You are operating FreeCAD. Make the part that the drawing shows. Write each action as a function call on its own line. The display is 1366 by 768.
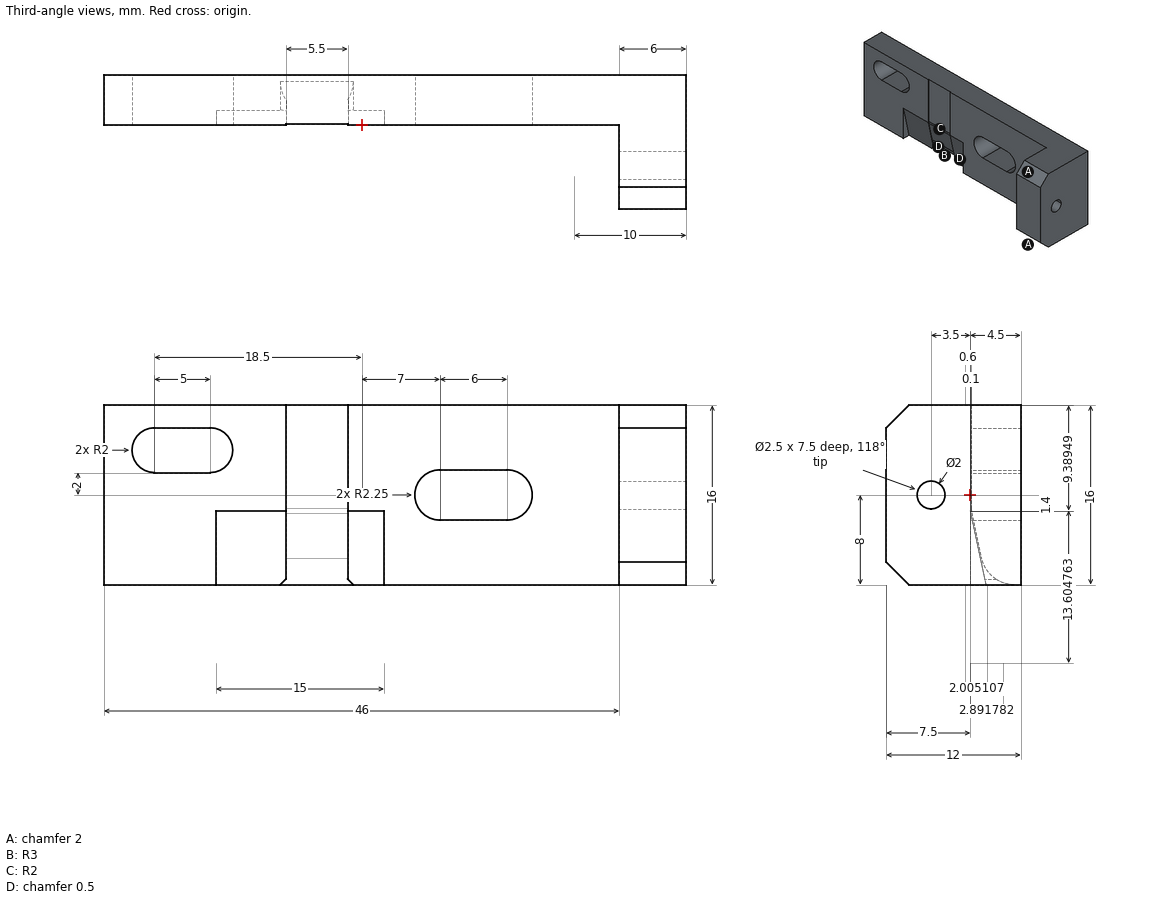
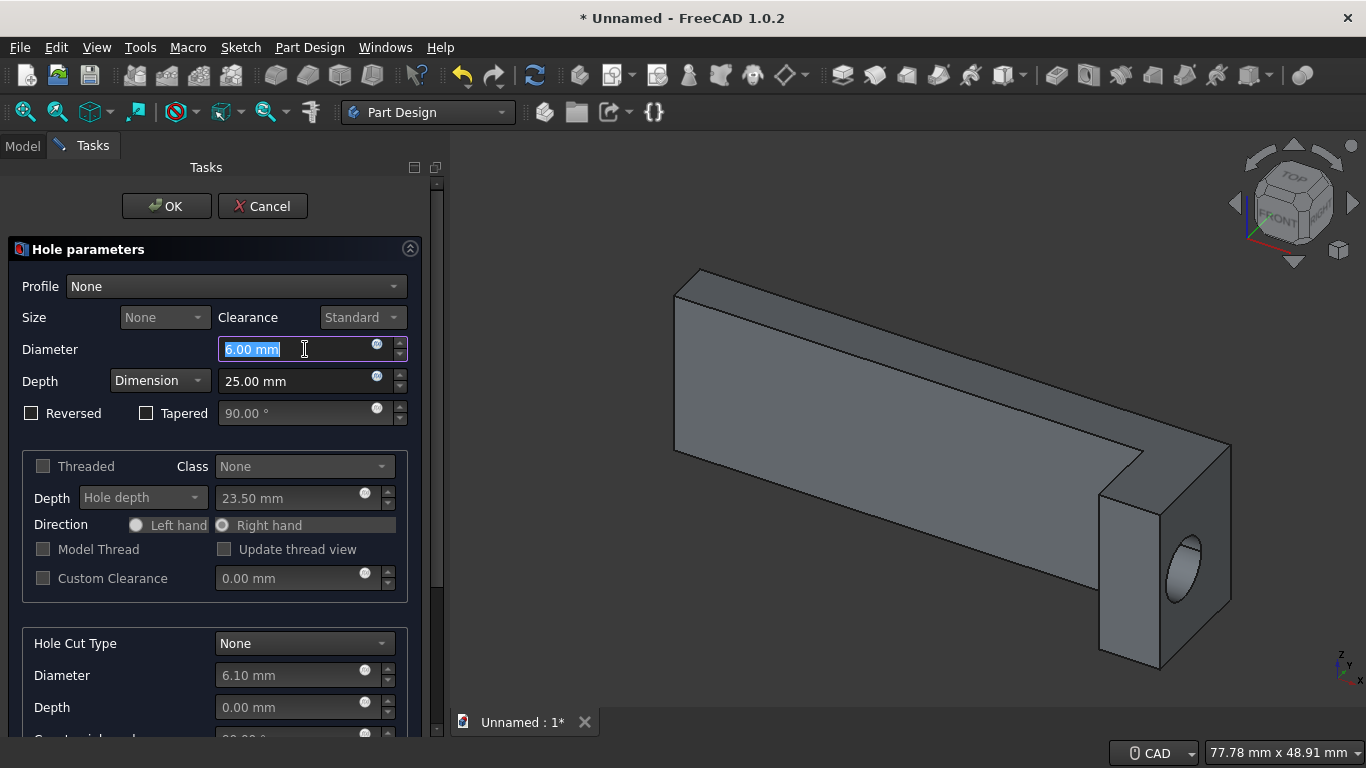
text(2.5)
key(Tab)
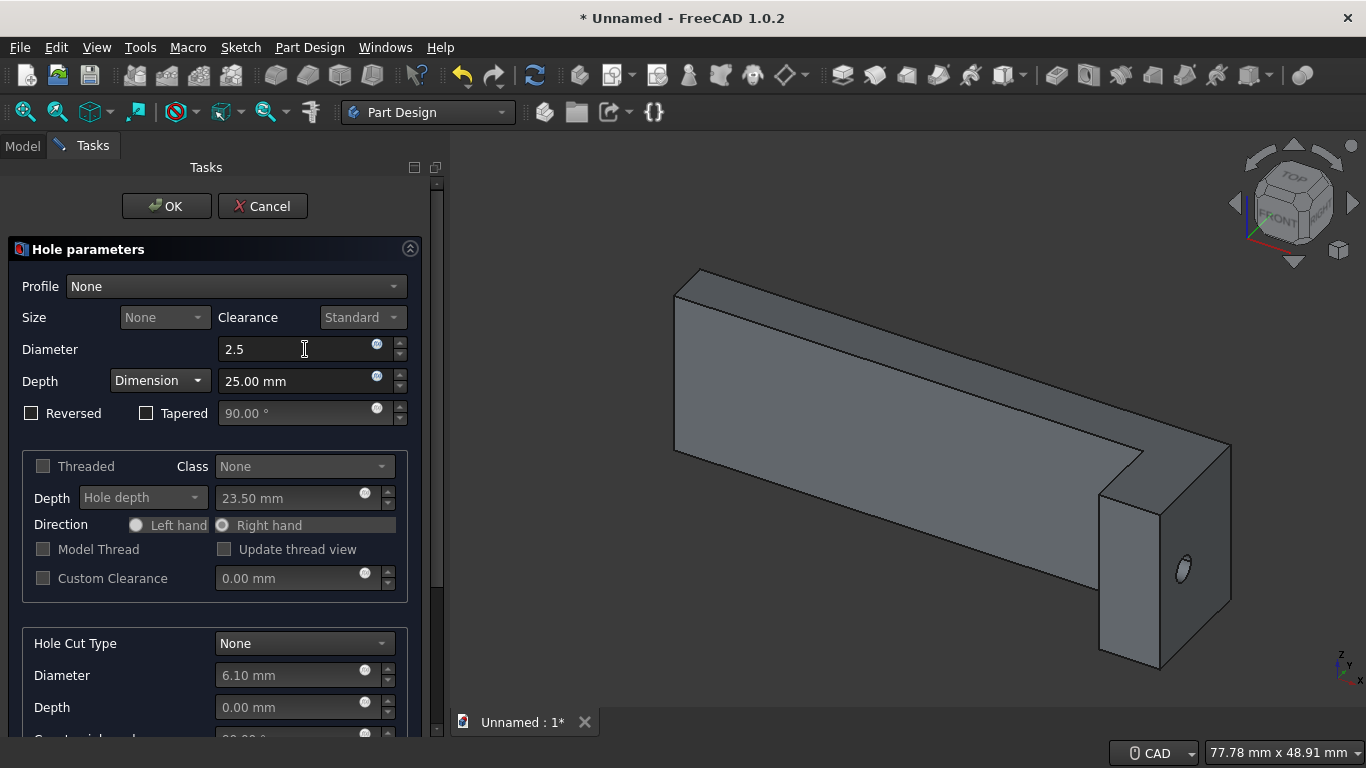
triple_click(305, 381)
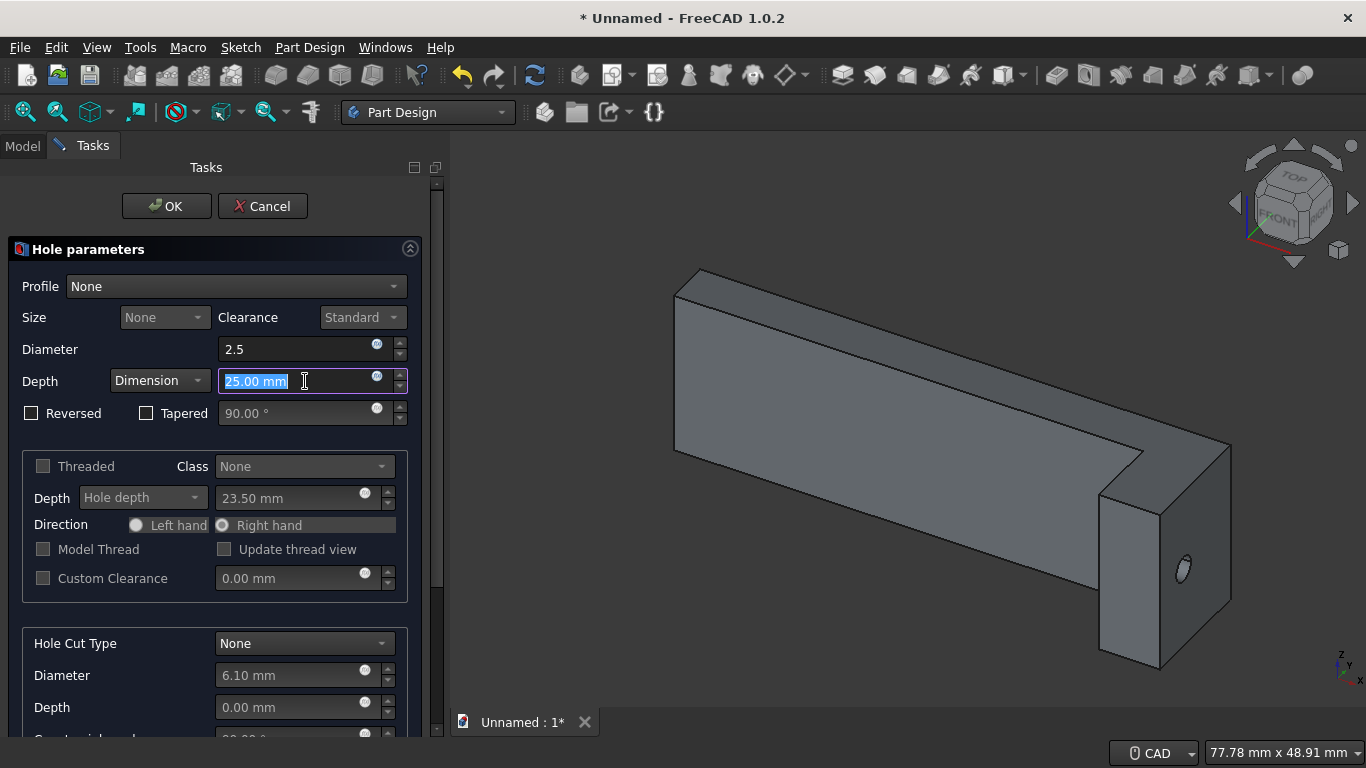
text(7.5)
key(Tab)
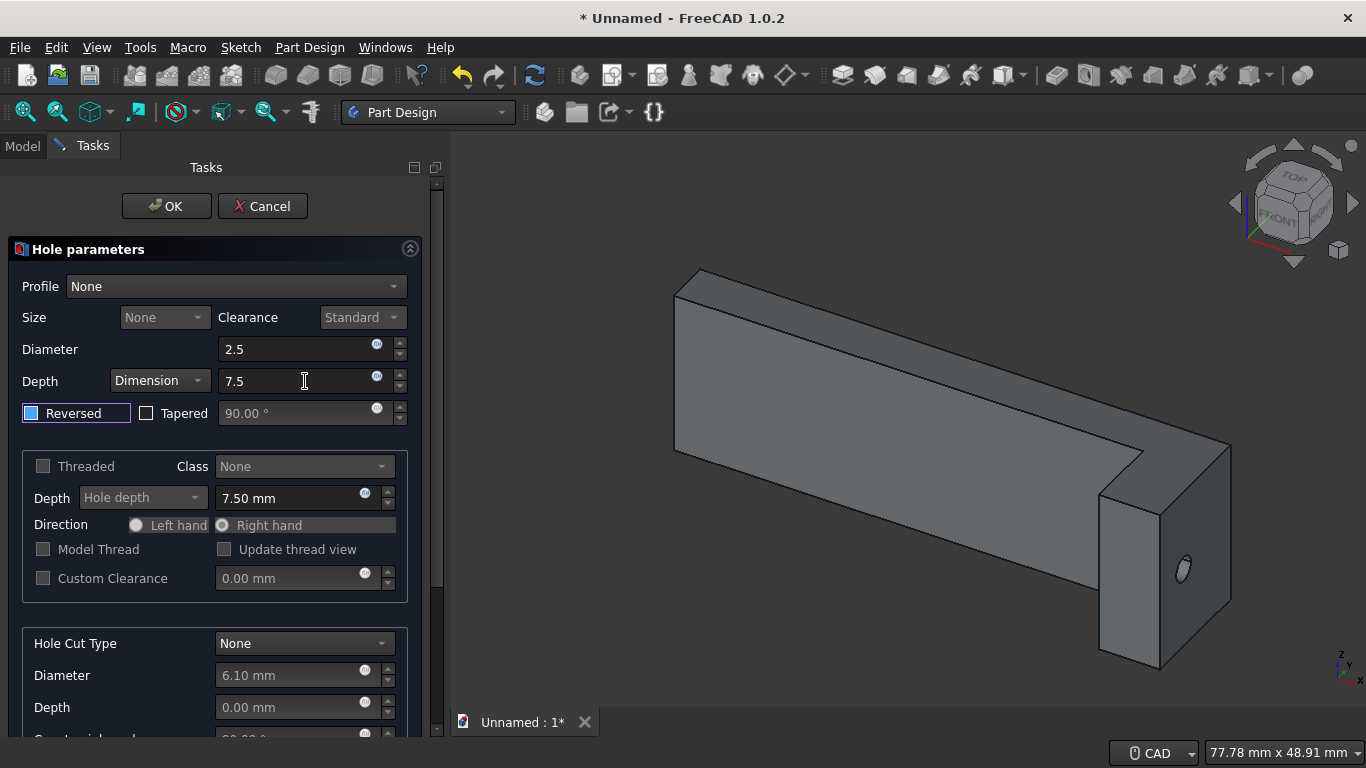
click(167, 206)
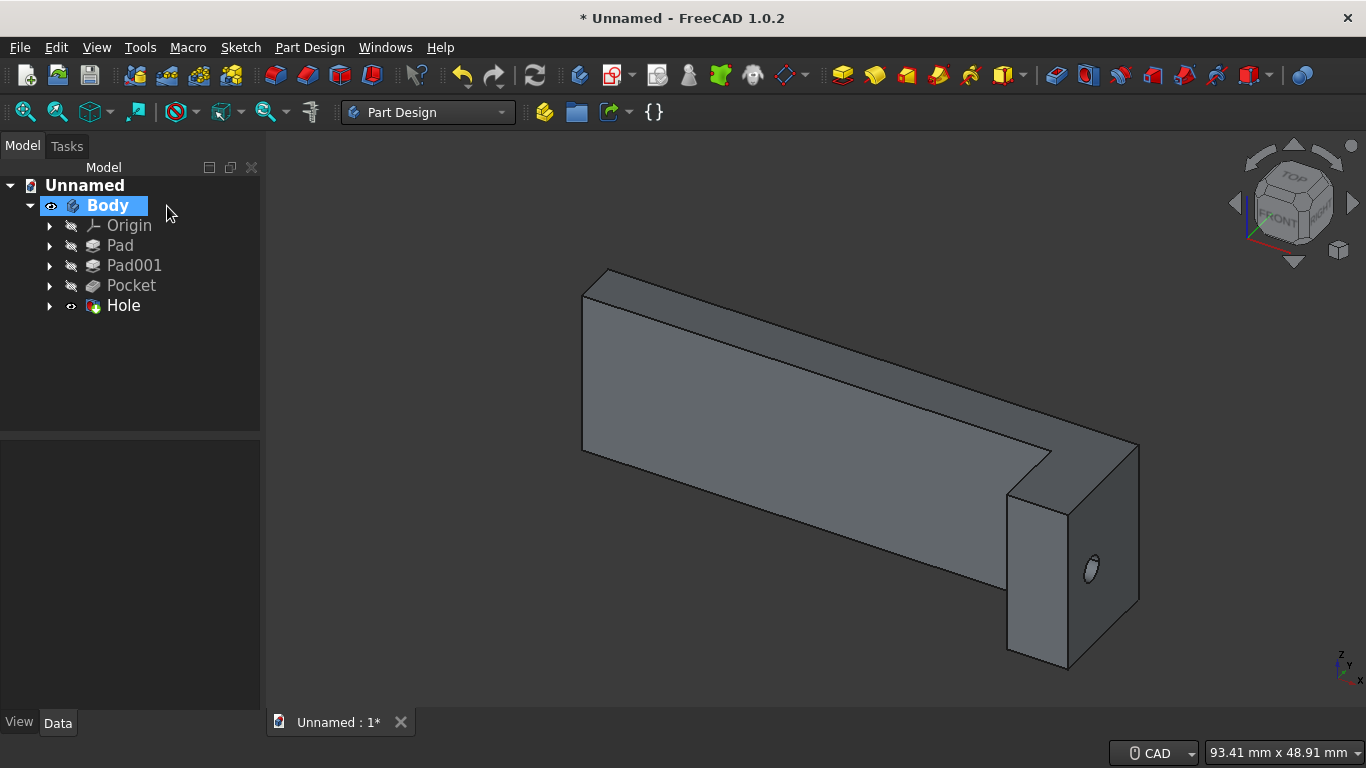
click(1037, 504)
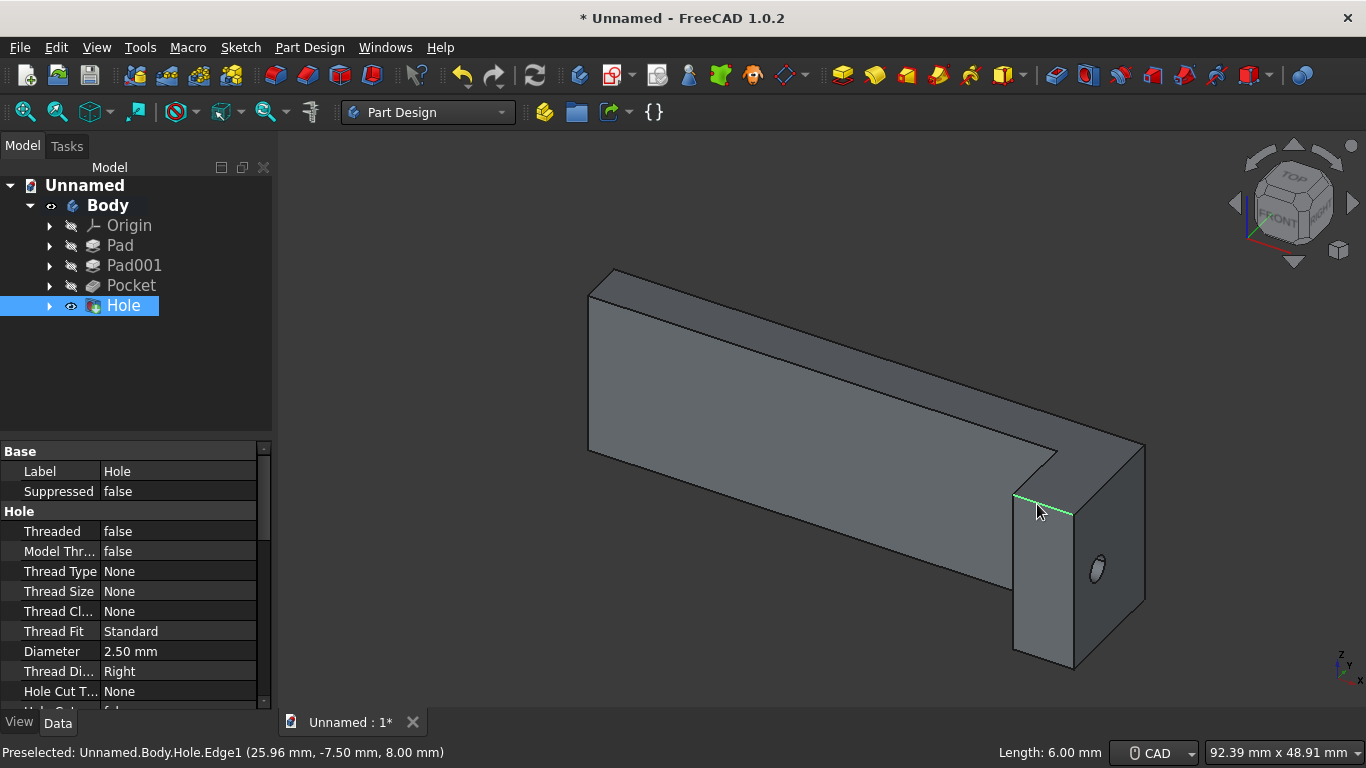
key(0)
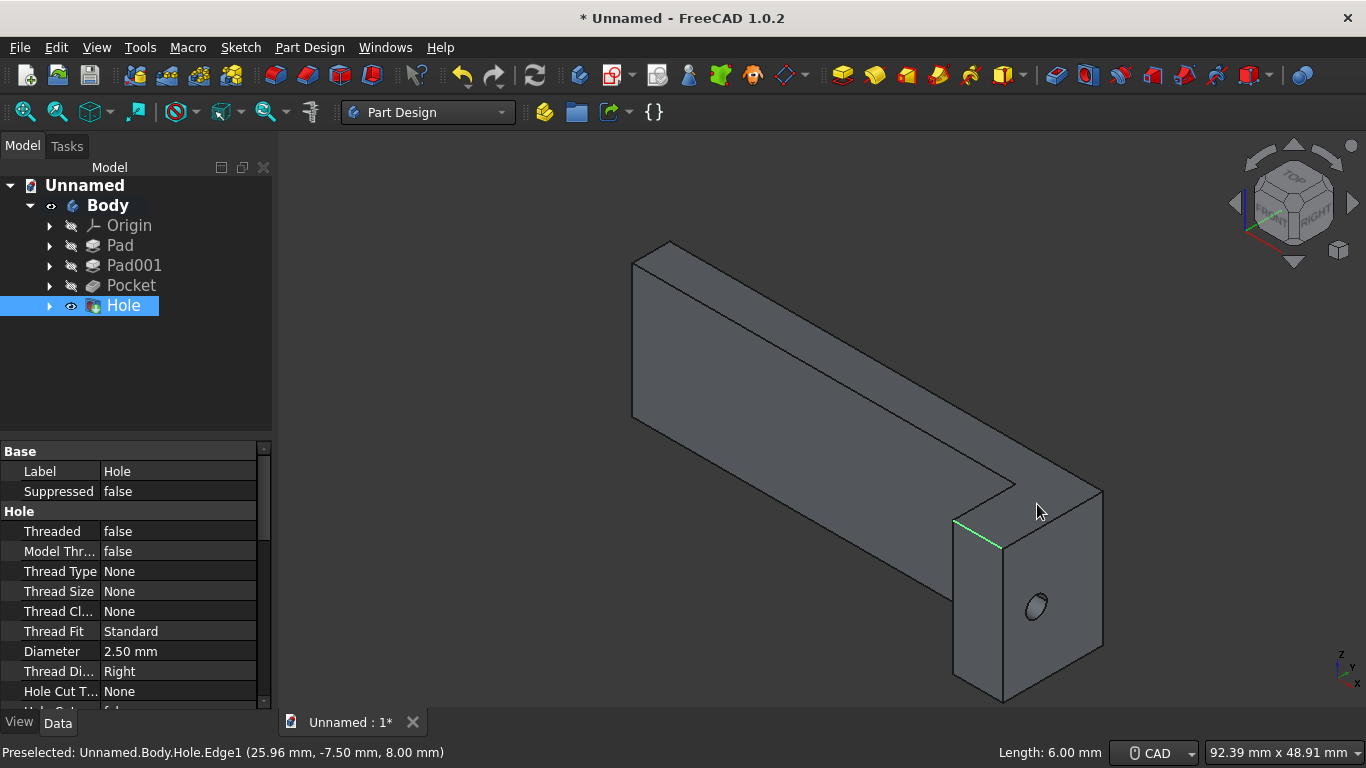
key(2)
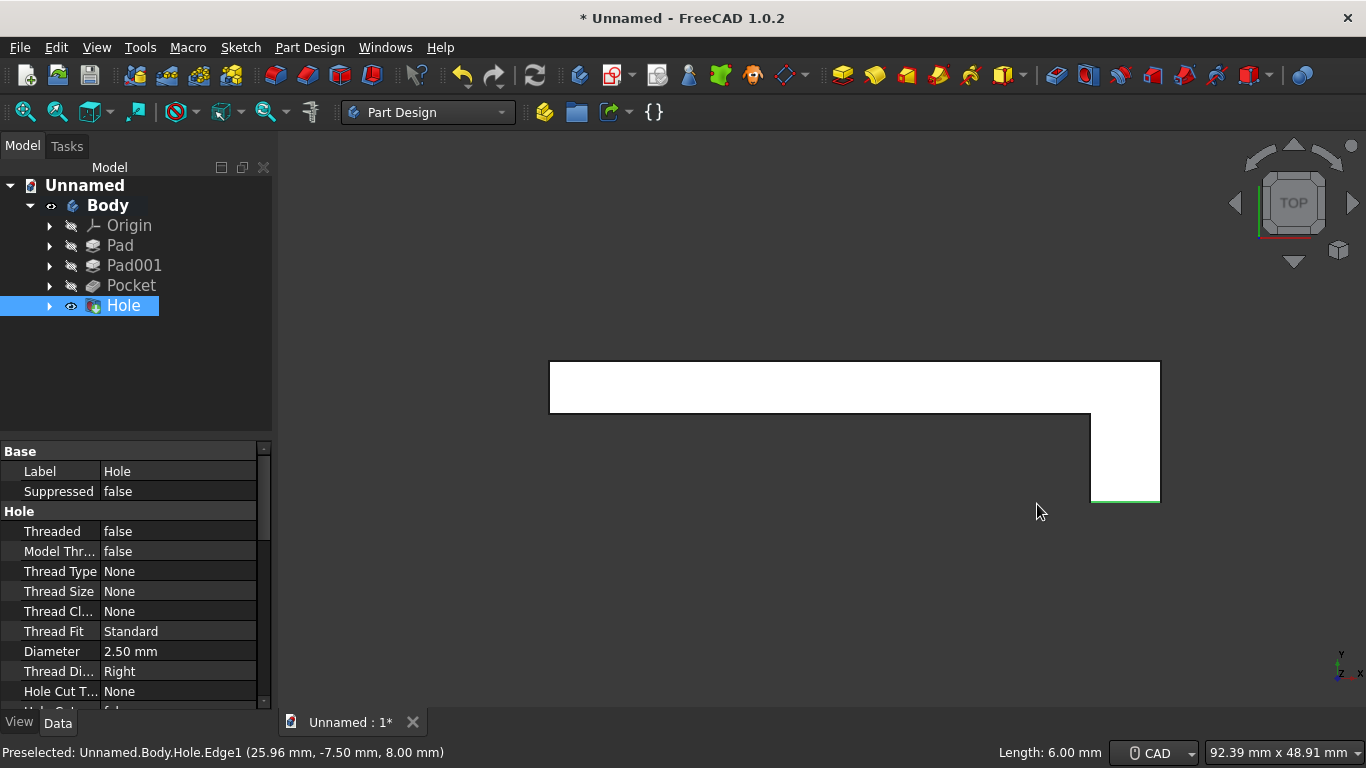
key(1)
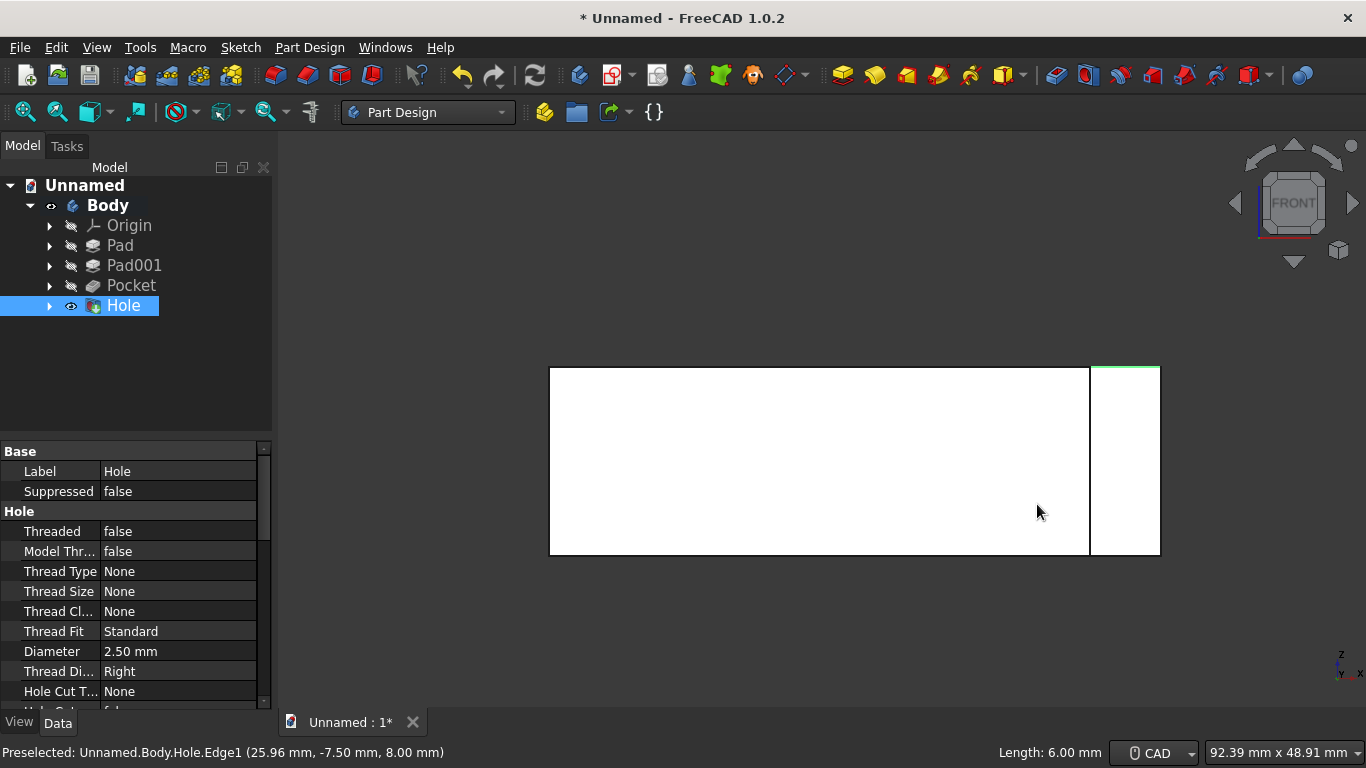
key(3)